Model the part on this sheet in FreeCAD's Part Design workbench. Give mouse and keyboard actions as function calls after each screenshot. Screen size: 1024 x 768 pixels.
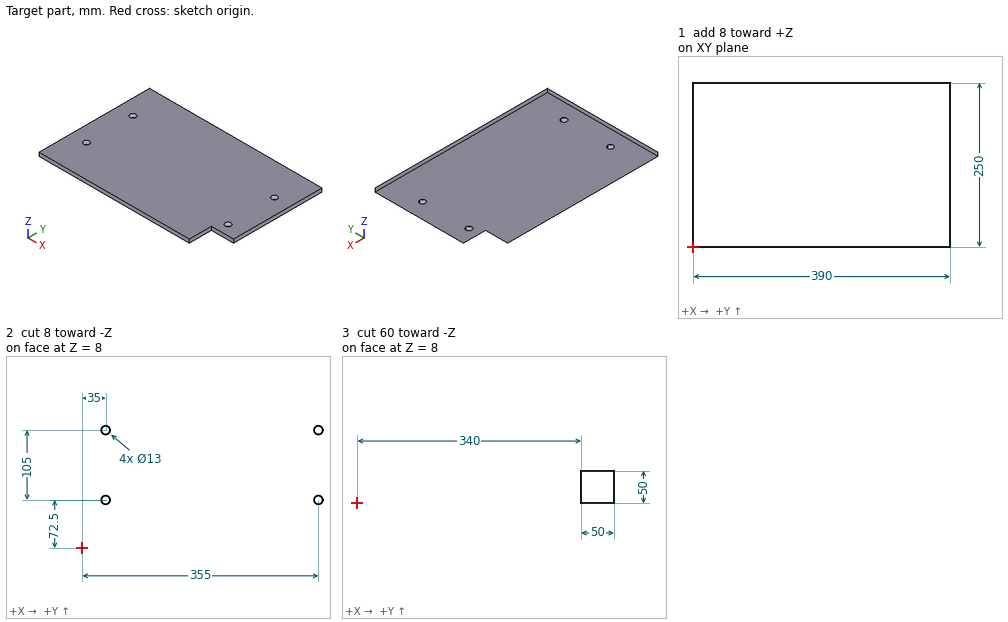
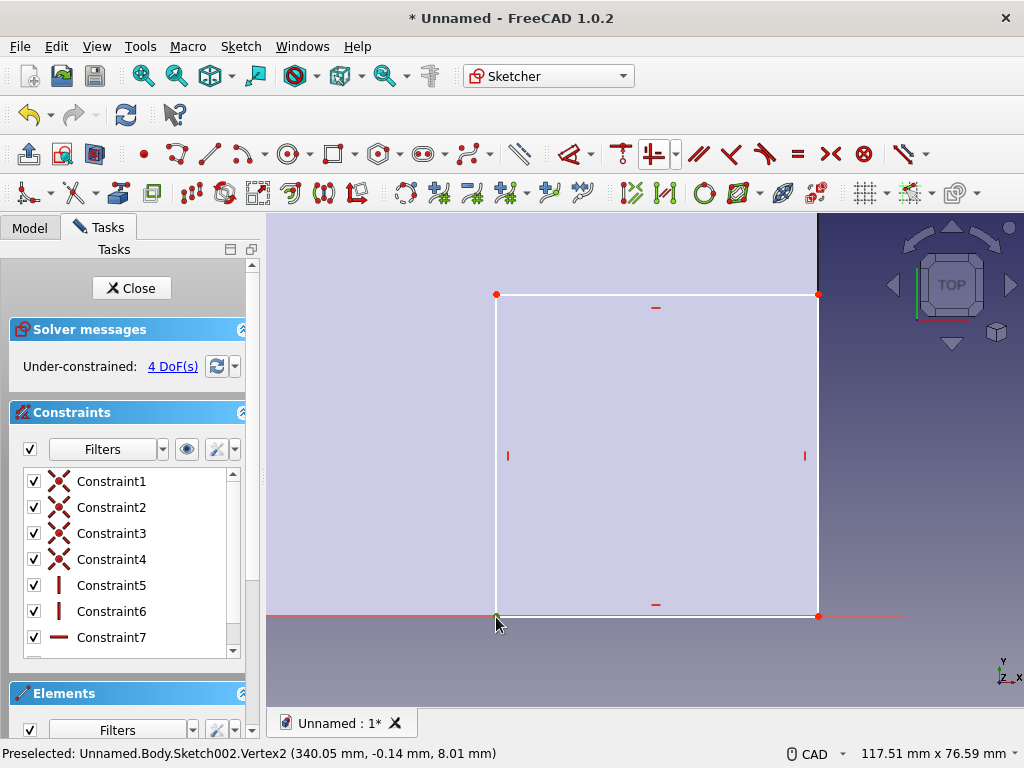
click(334, 616)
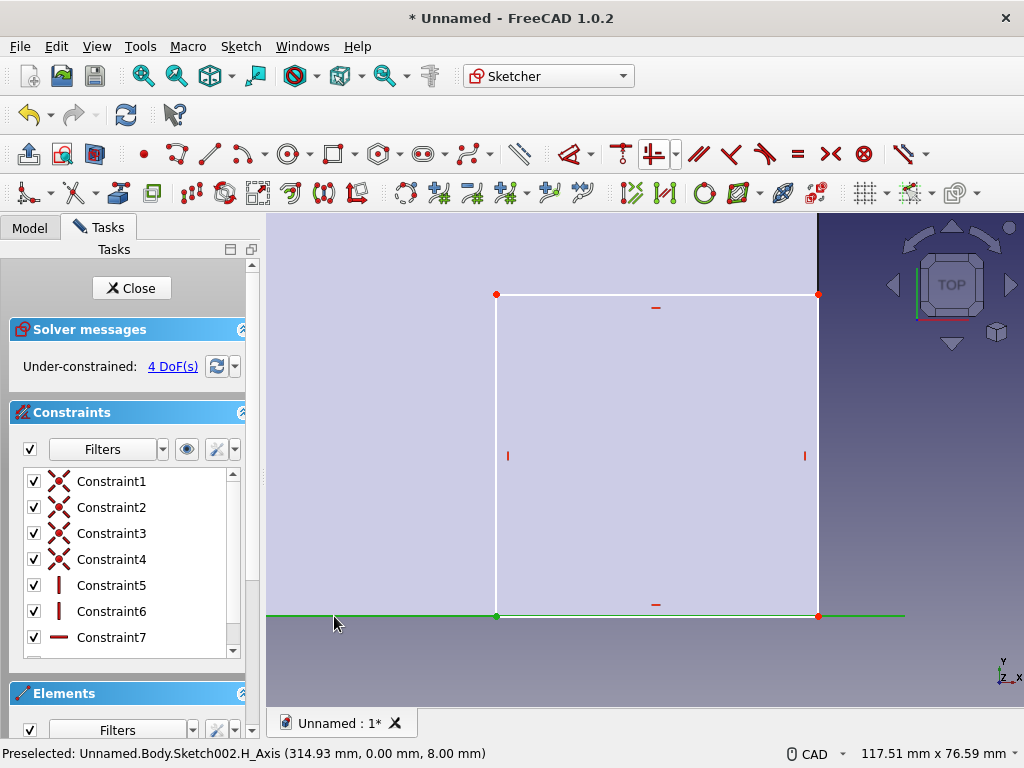
key(c)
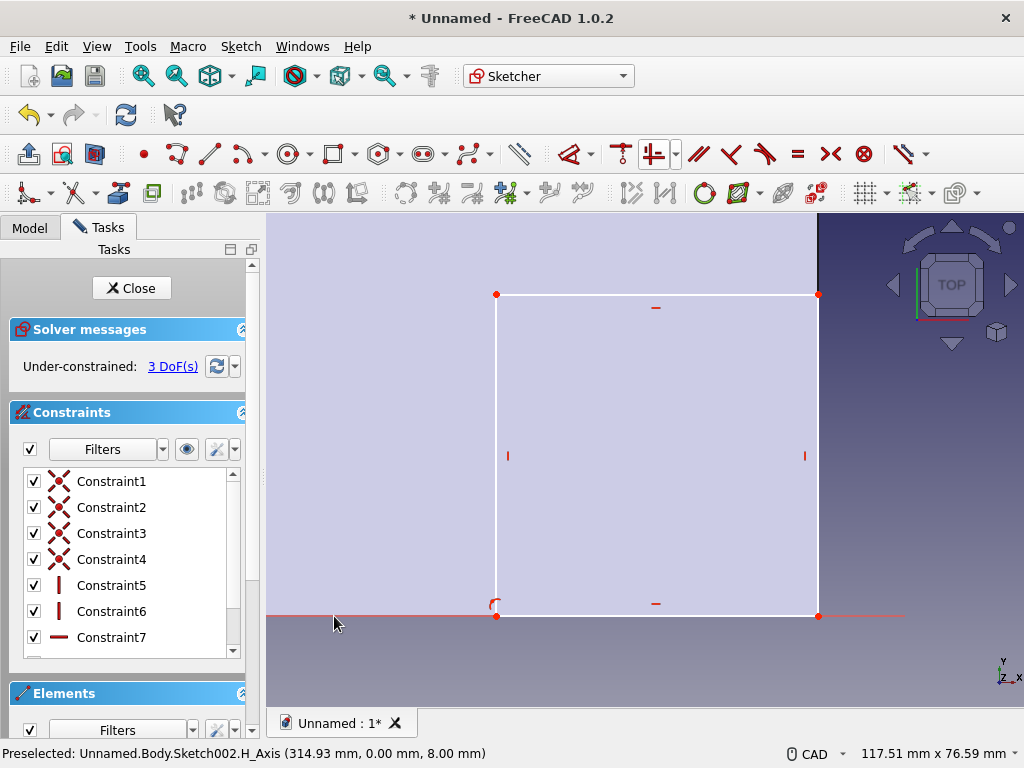
key(d)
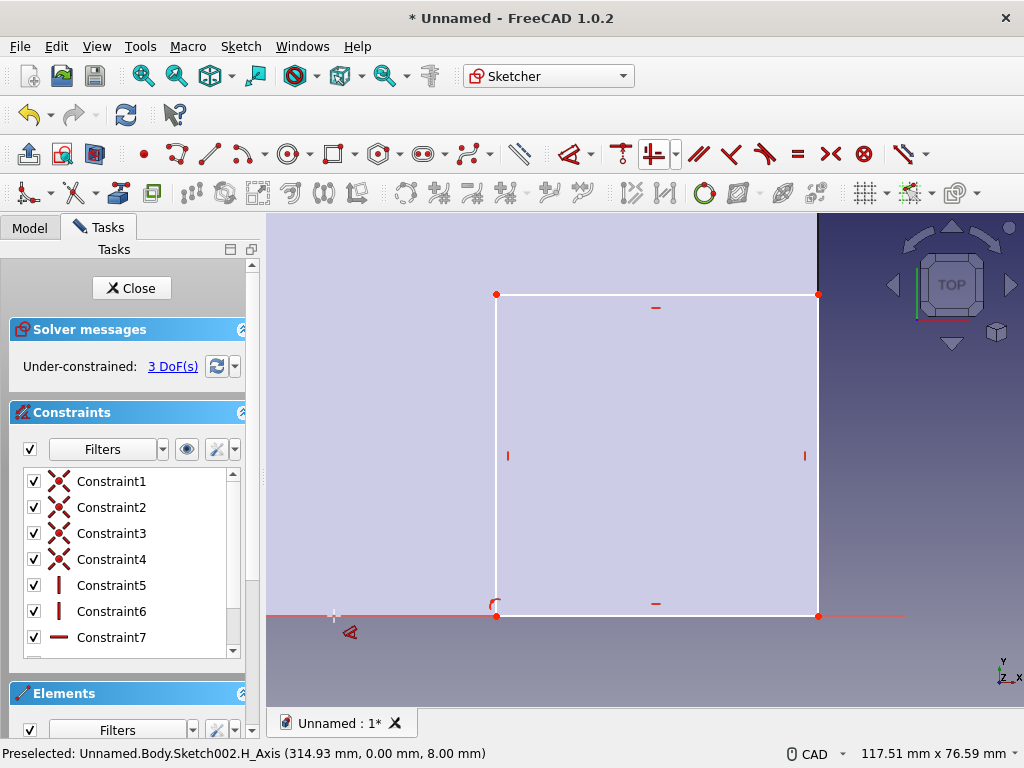
click(496, 391)
click(462, 456)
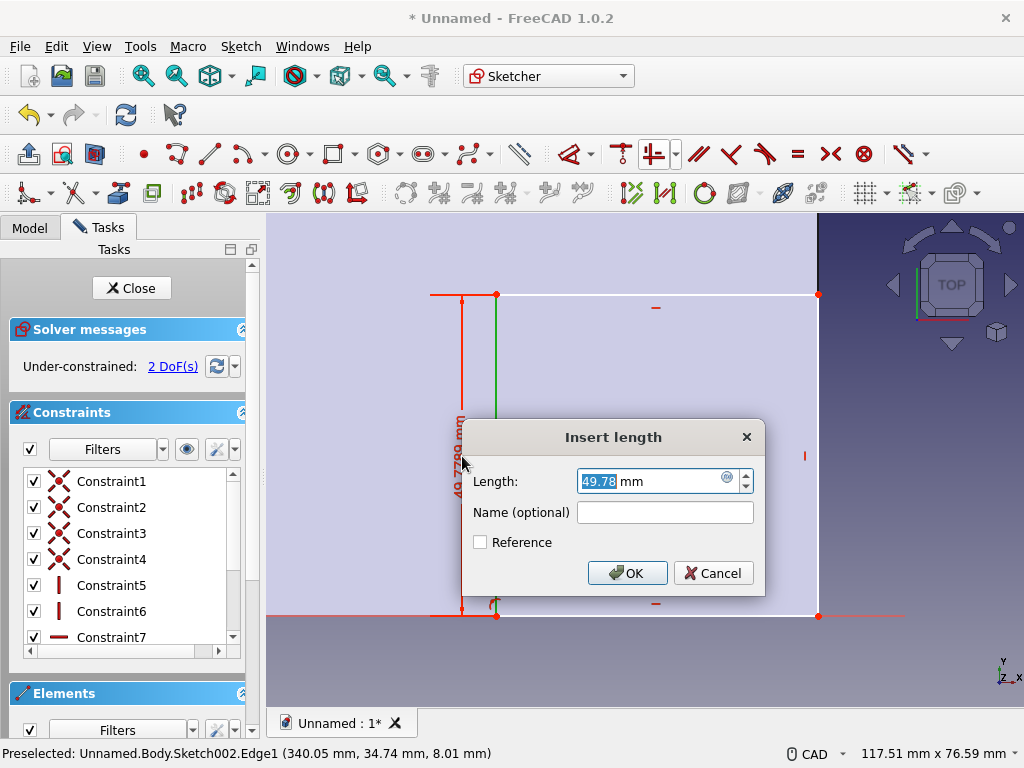
text(50)
key(Return)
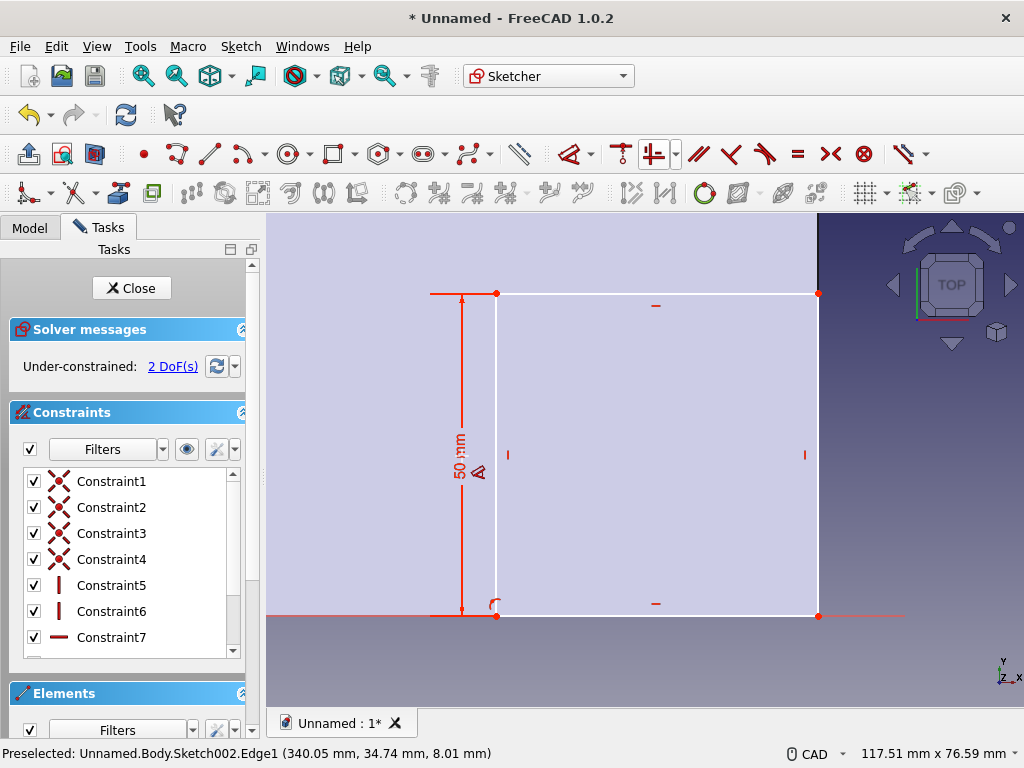
click(593, 616)
click(657, 650)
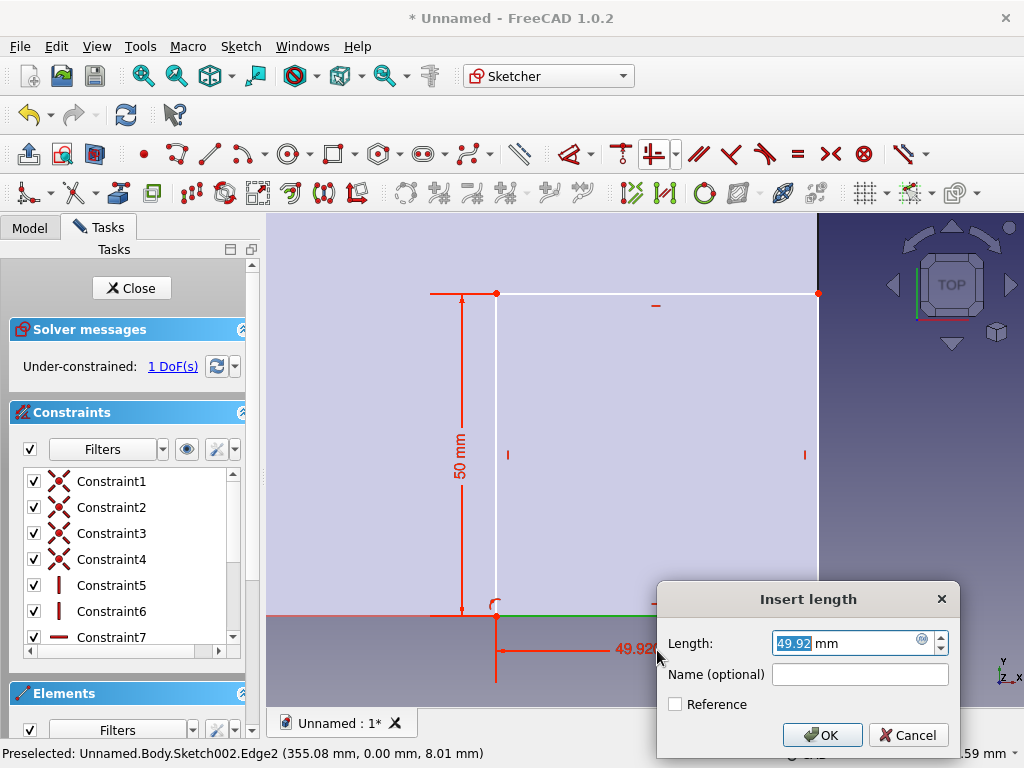
text(50)
key(Return)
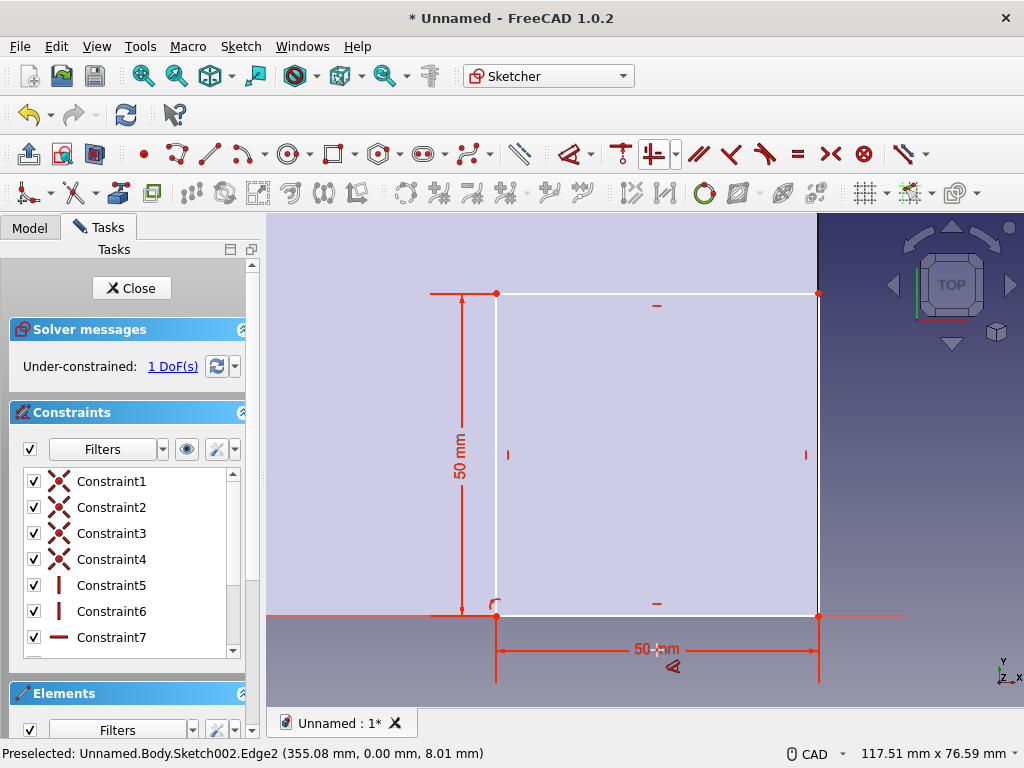
click(496, 294)
click(395, 650)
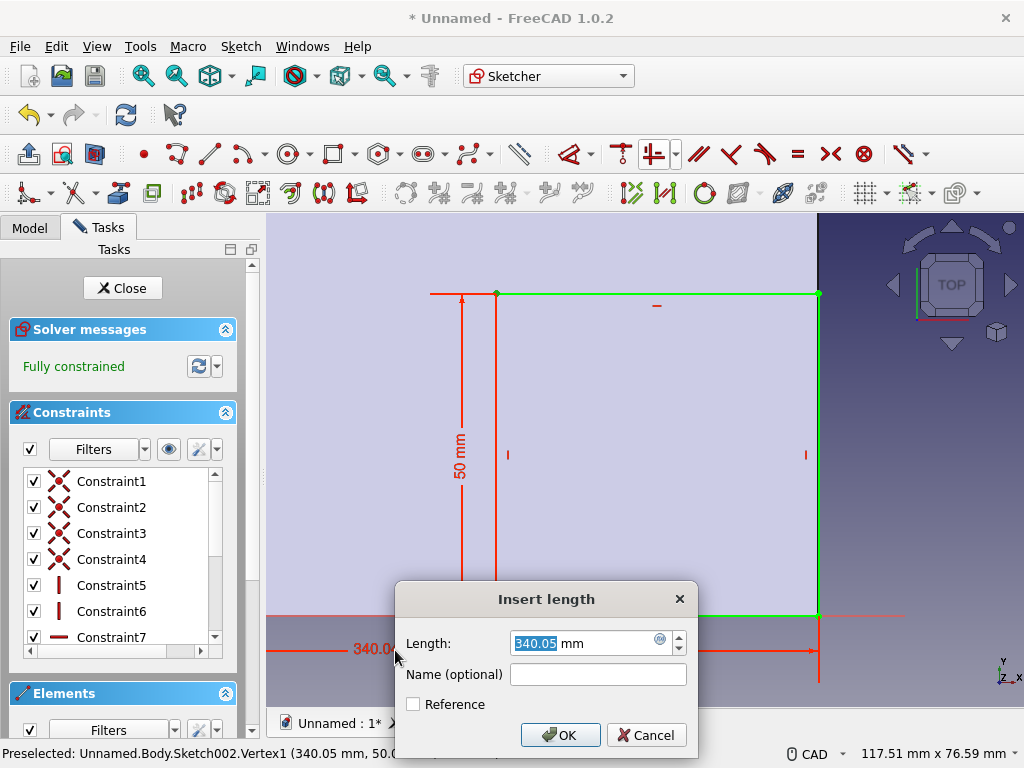
text(340)
key(Return)
key(Escape)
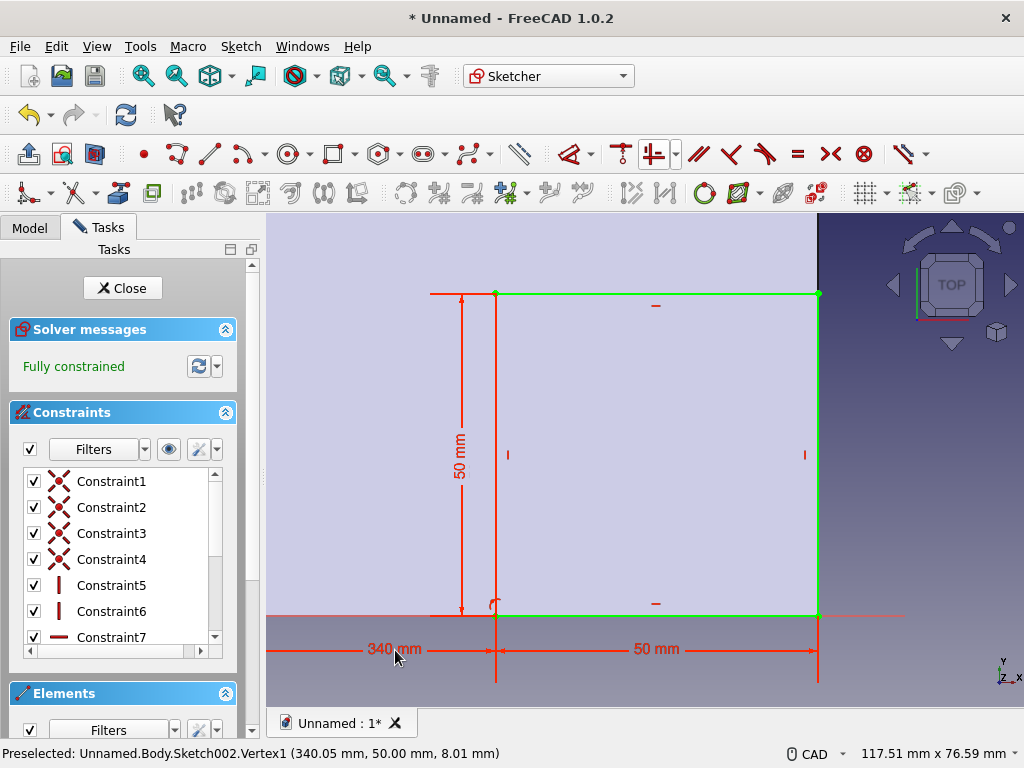
click(123, 288)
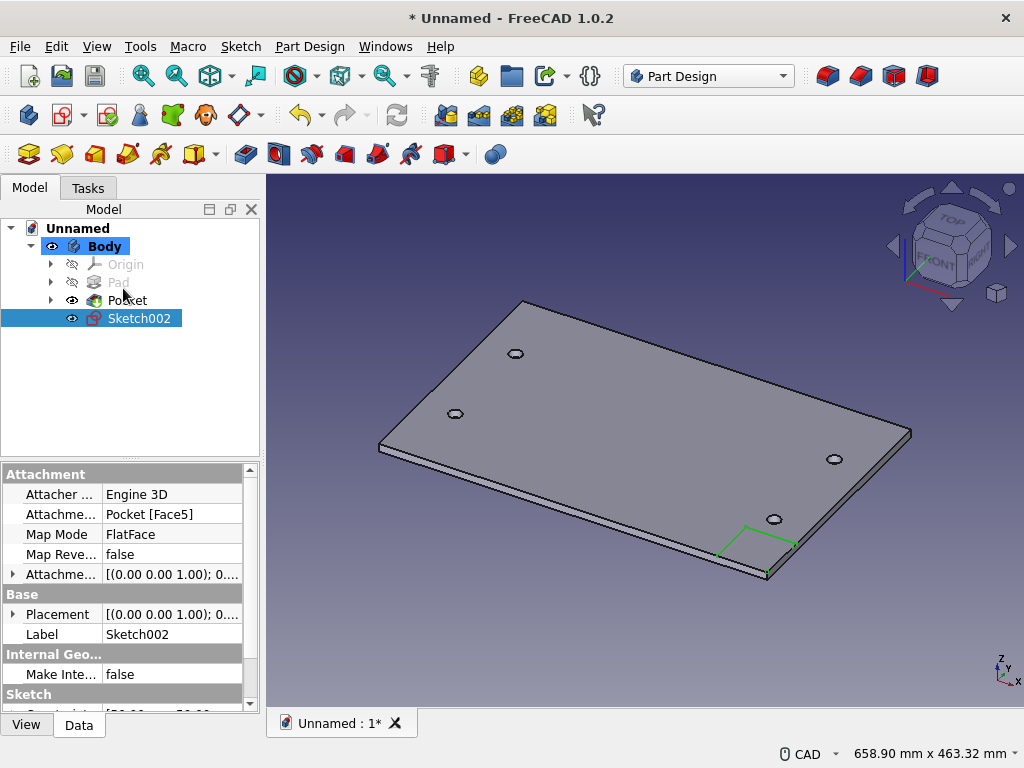
click(246, 154)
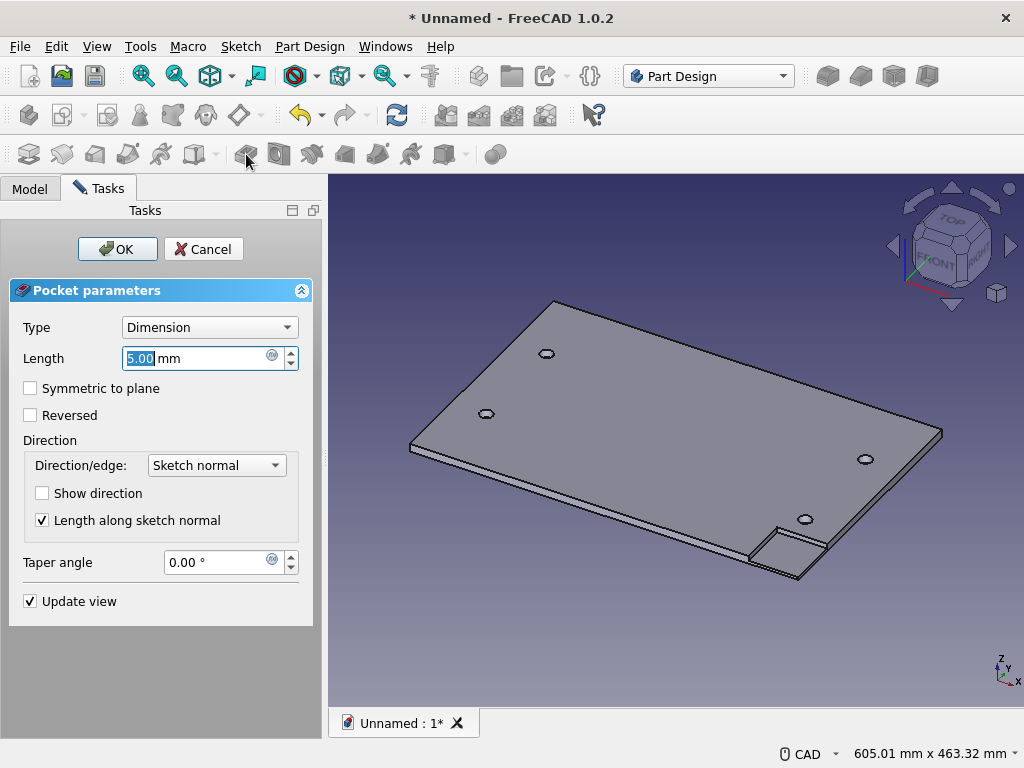
text(60)
key(Tab)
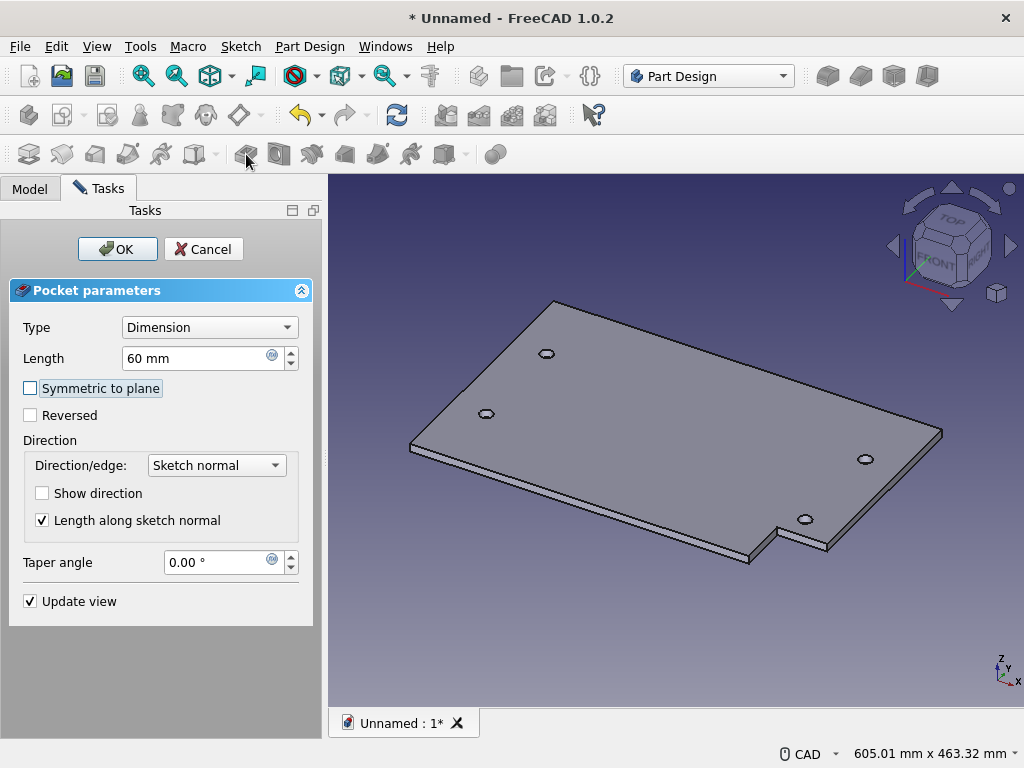
click(118, 249)